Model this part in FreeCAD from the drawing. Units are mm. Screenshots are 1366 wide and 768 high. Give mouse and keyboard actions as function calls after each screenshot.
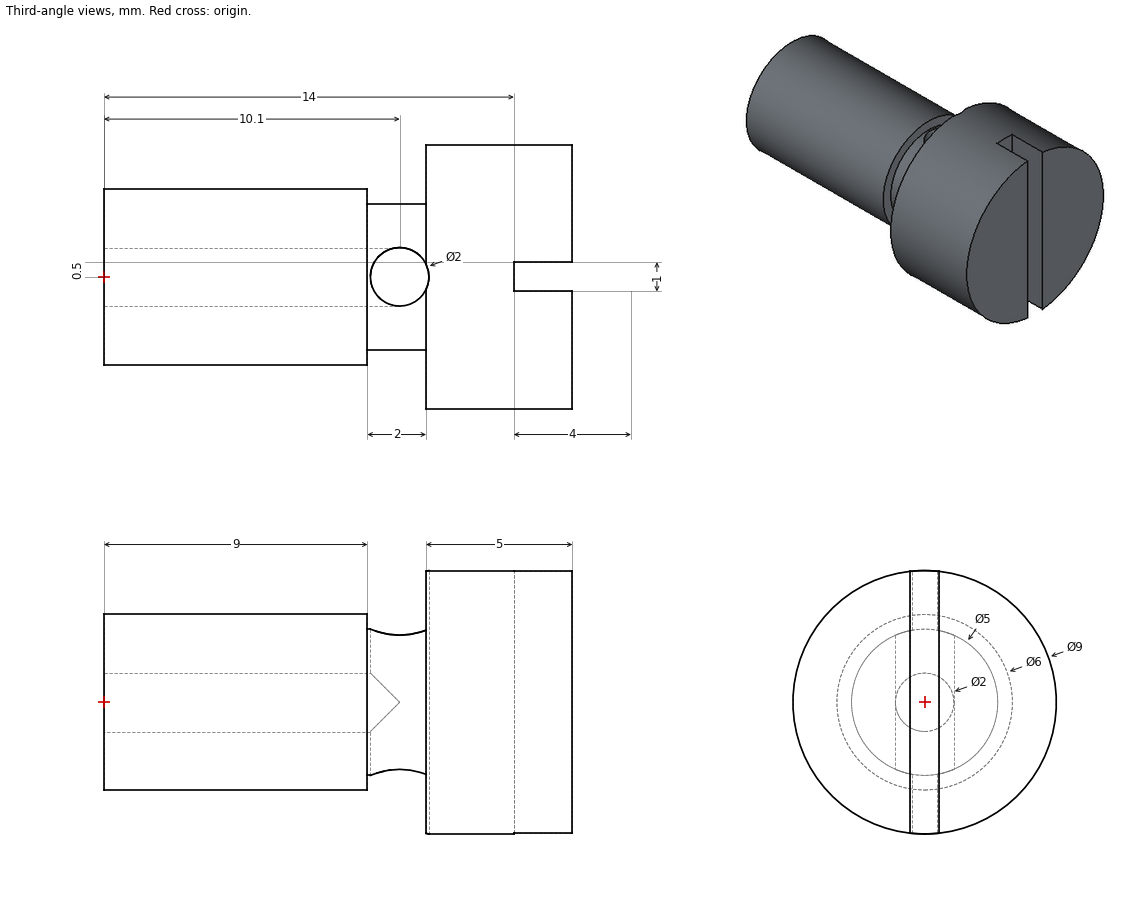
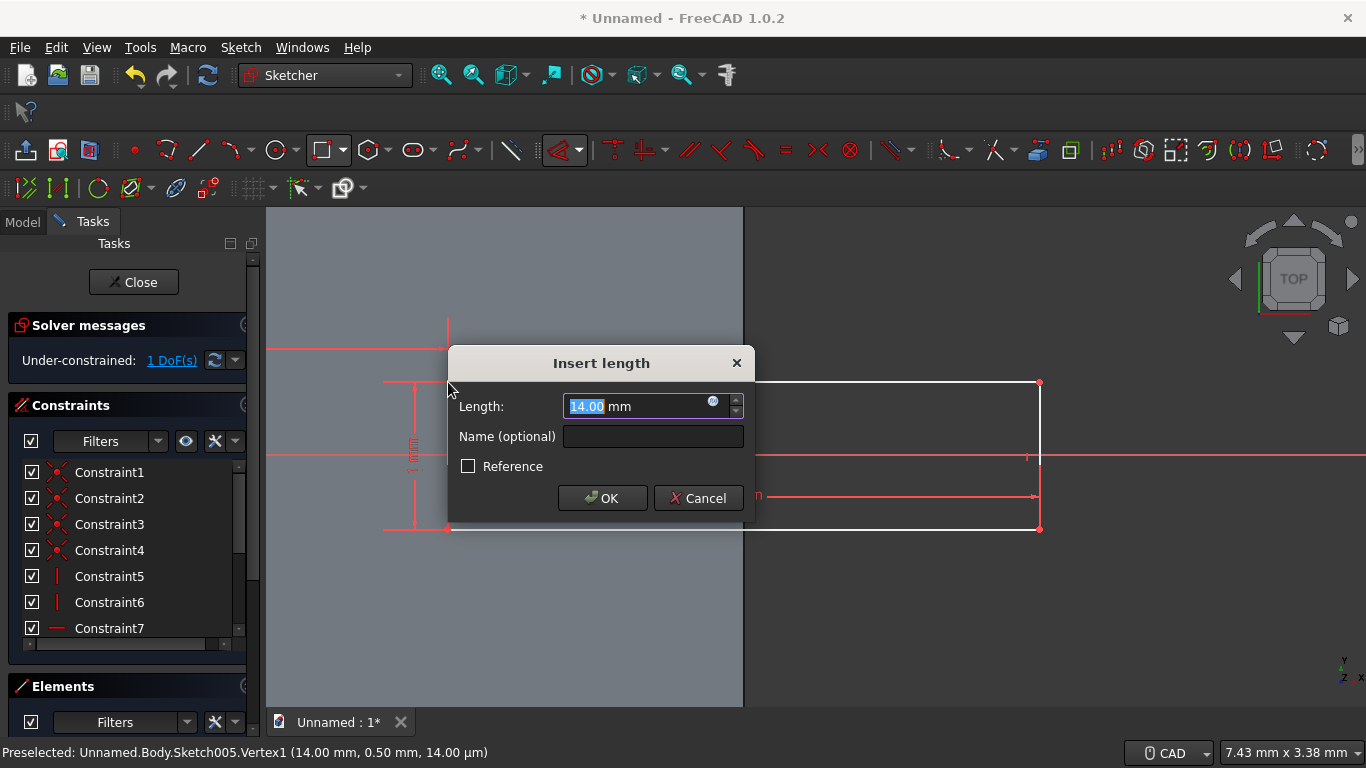
text(14)
key(Return)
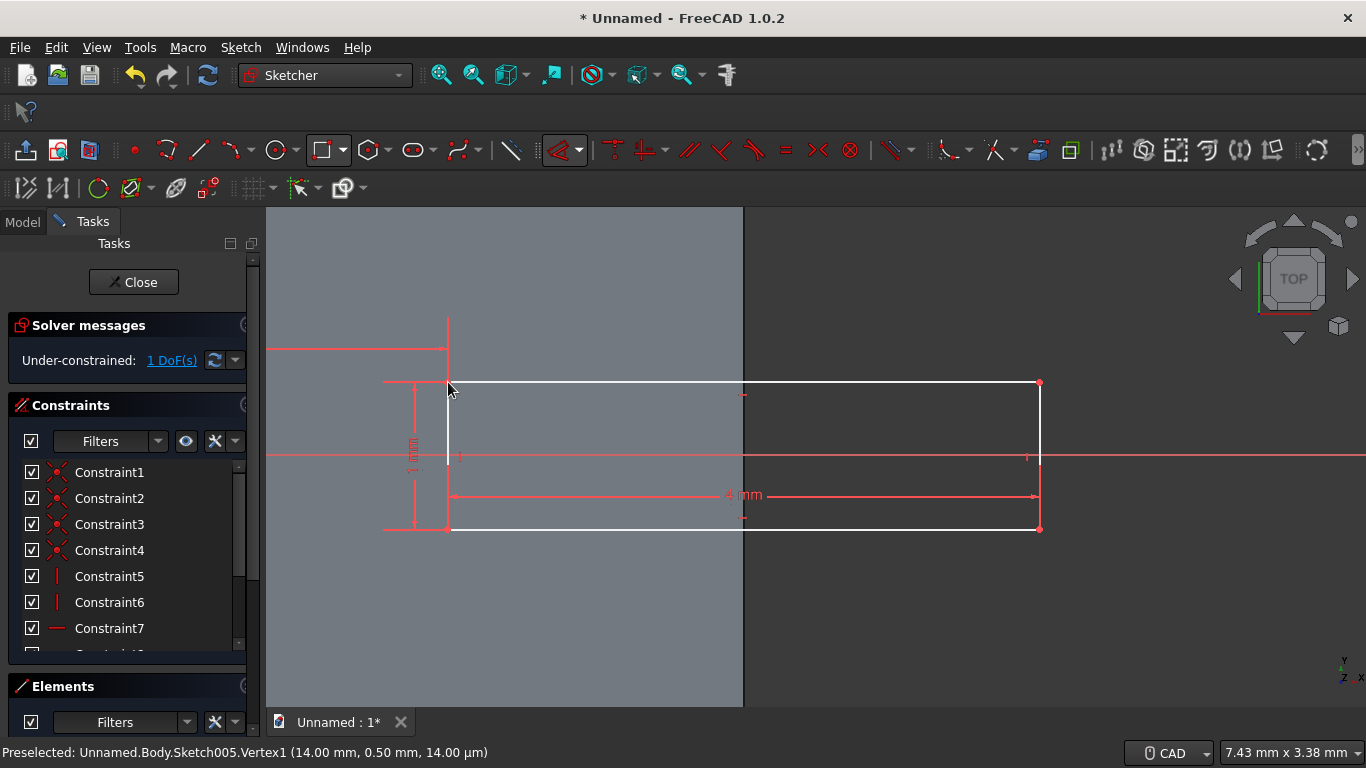
click(448, 382)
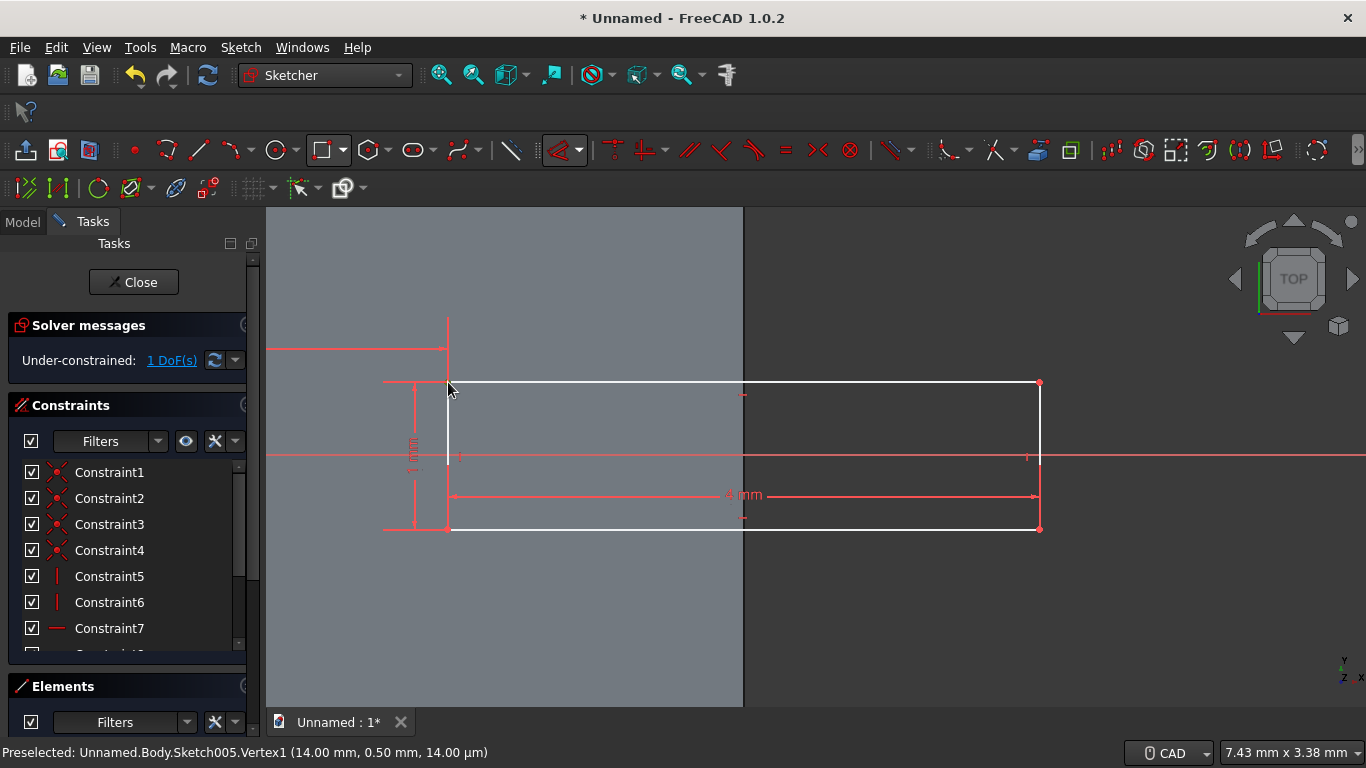
click(582, 150)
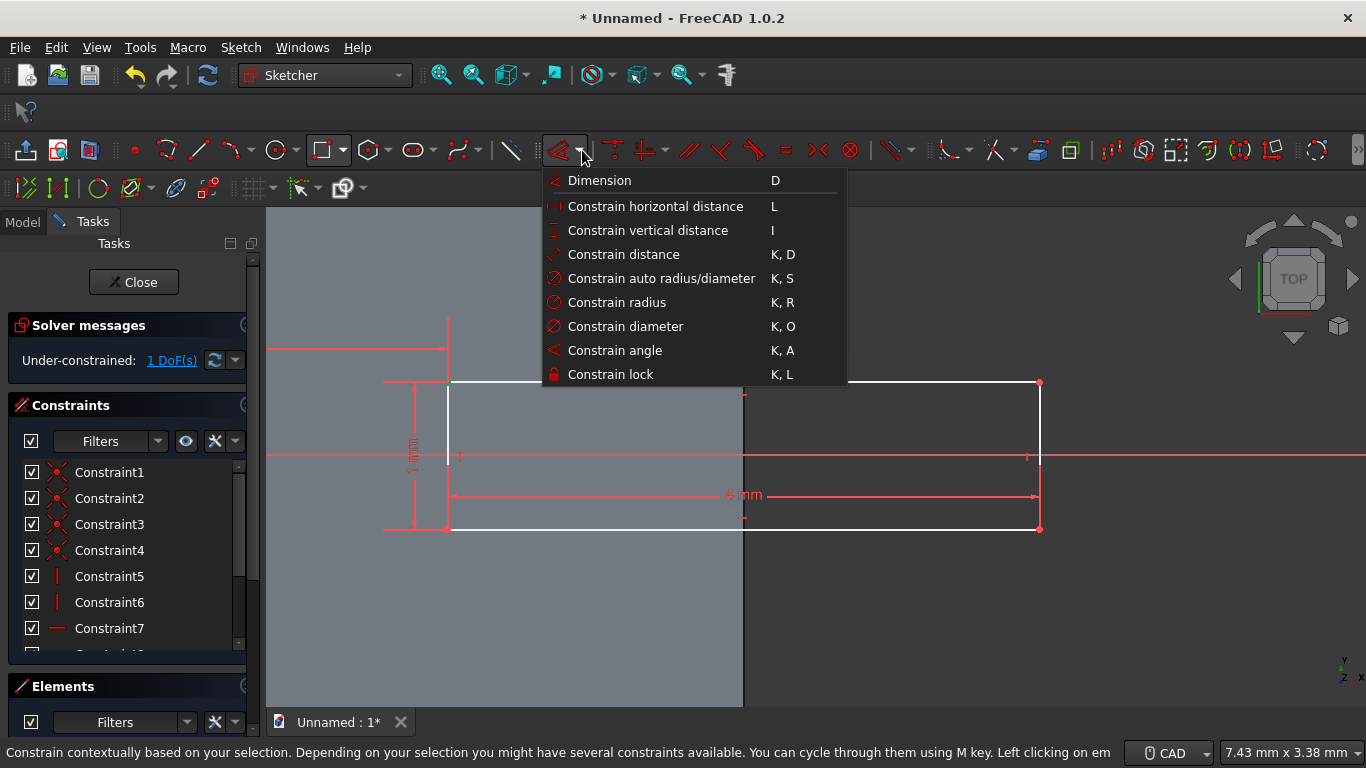
click(695, 230)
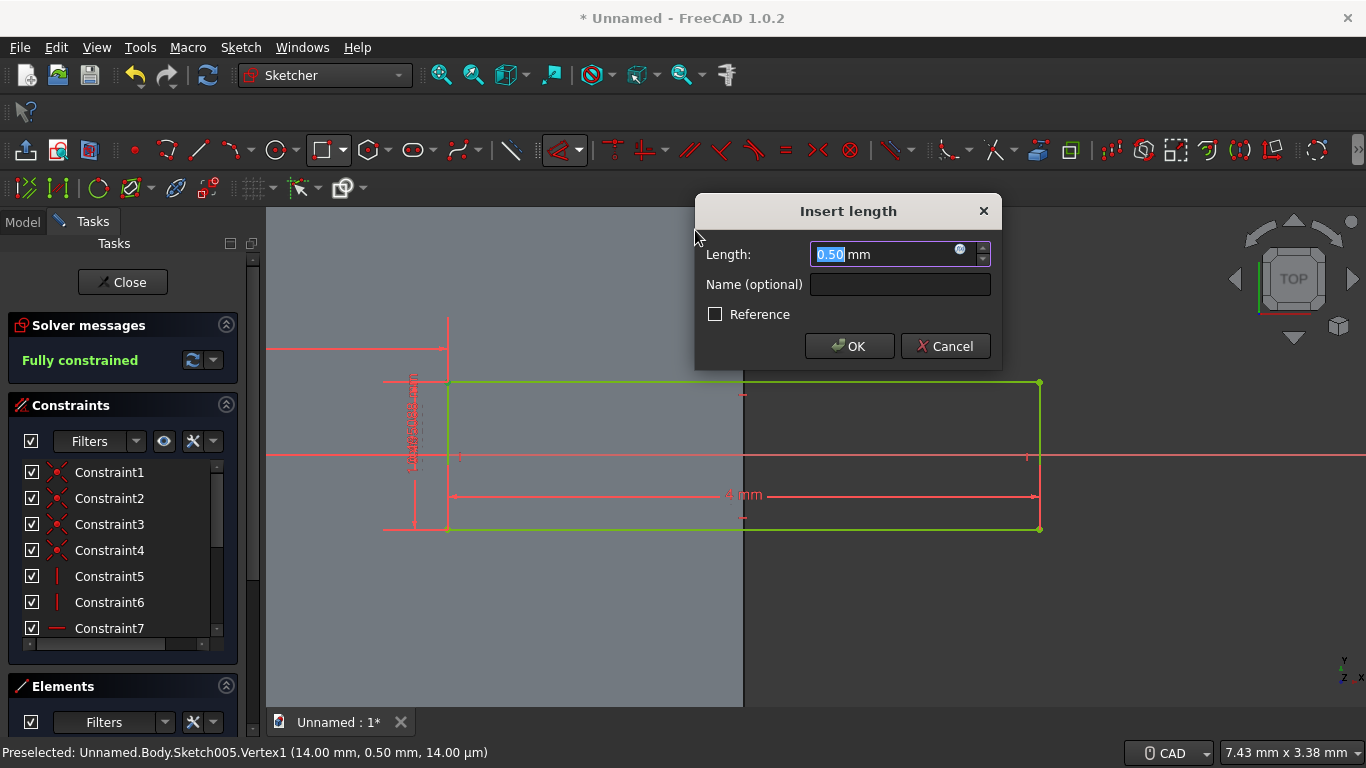
text(0.5)
key(Return)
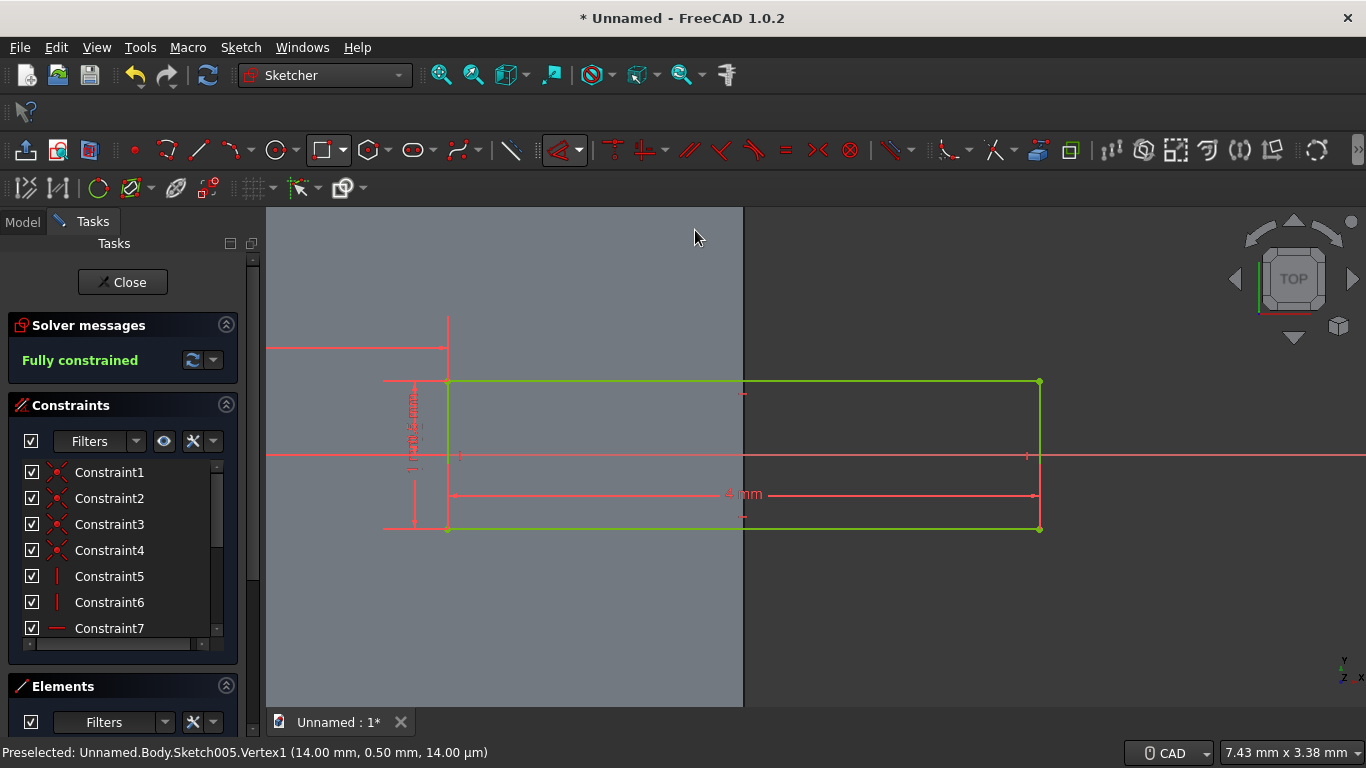
click(123, 282)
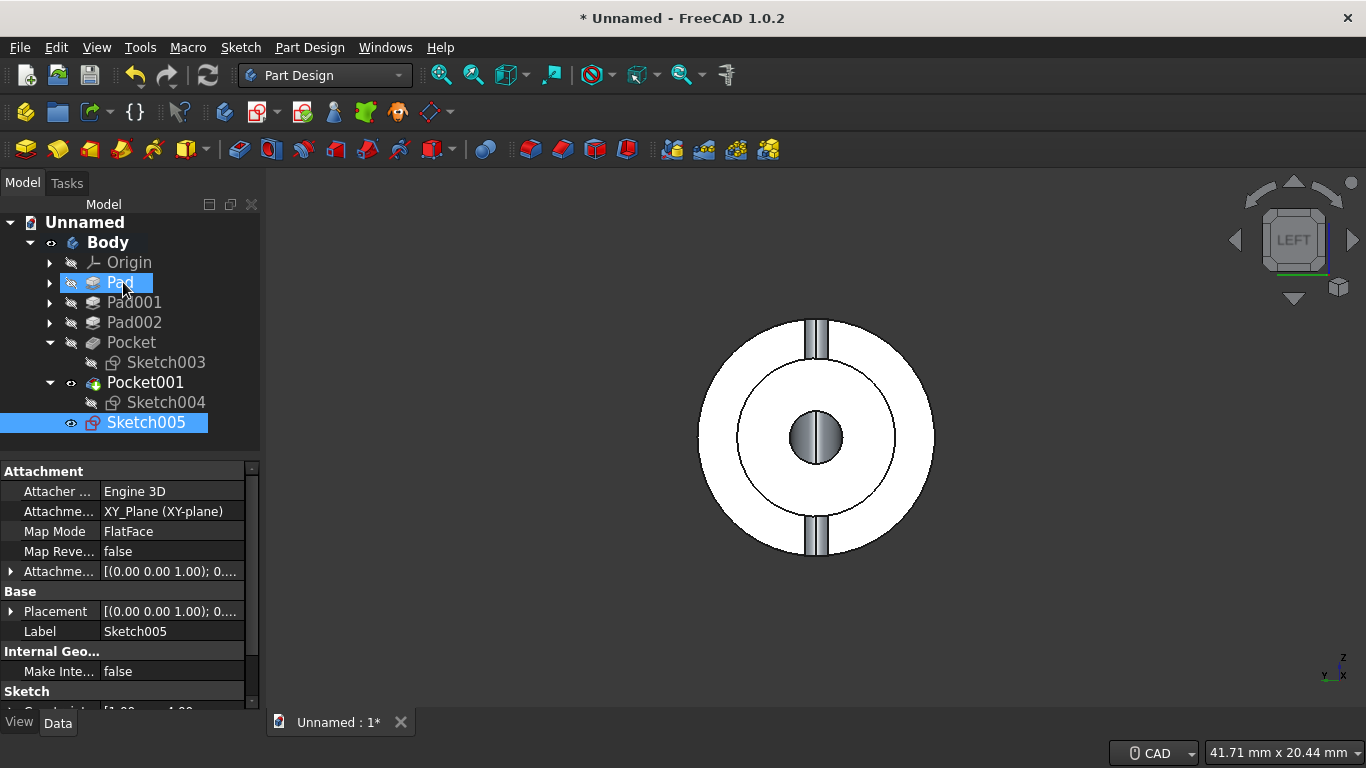
click(240, 150)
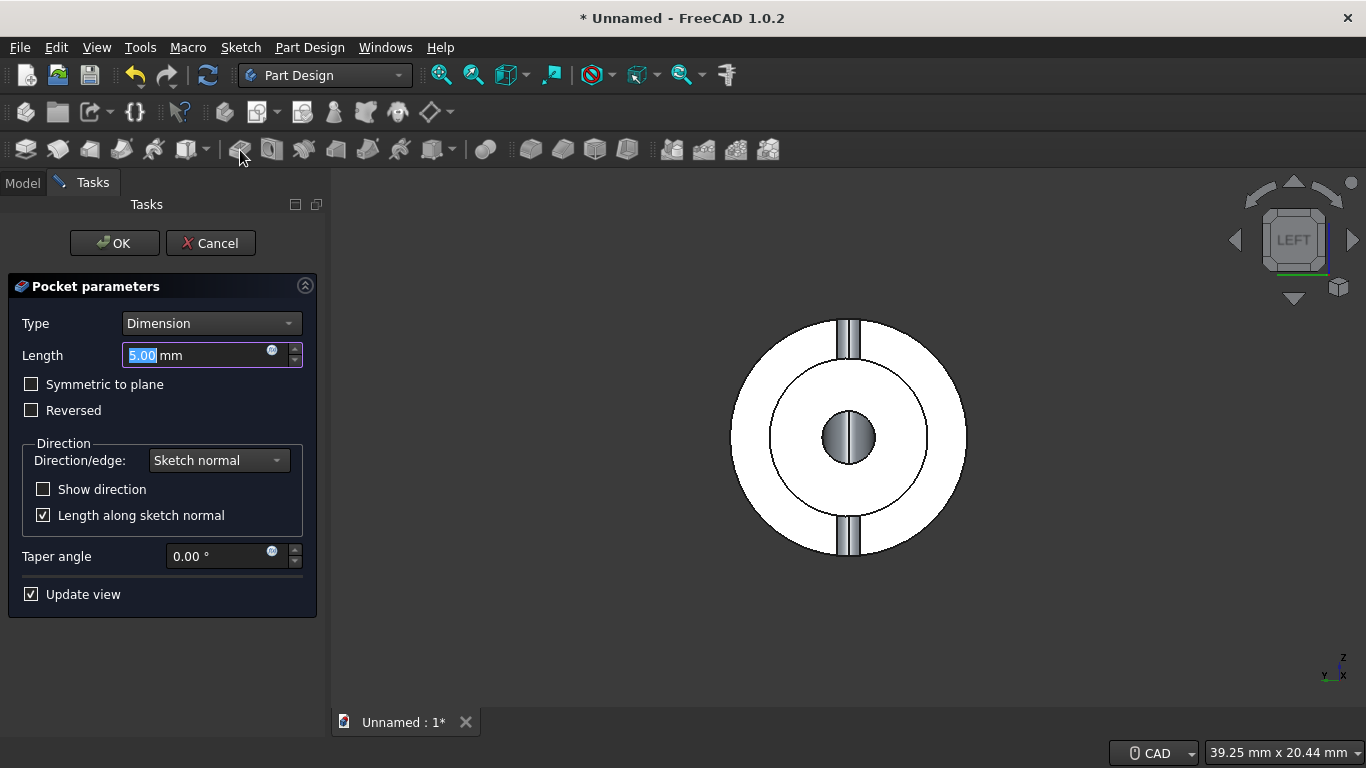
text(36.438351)
key(Tab)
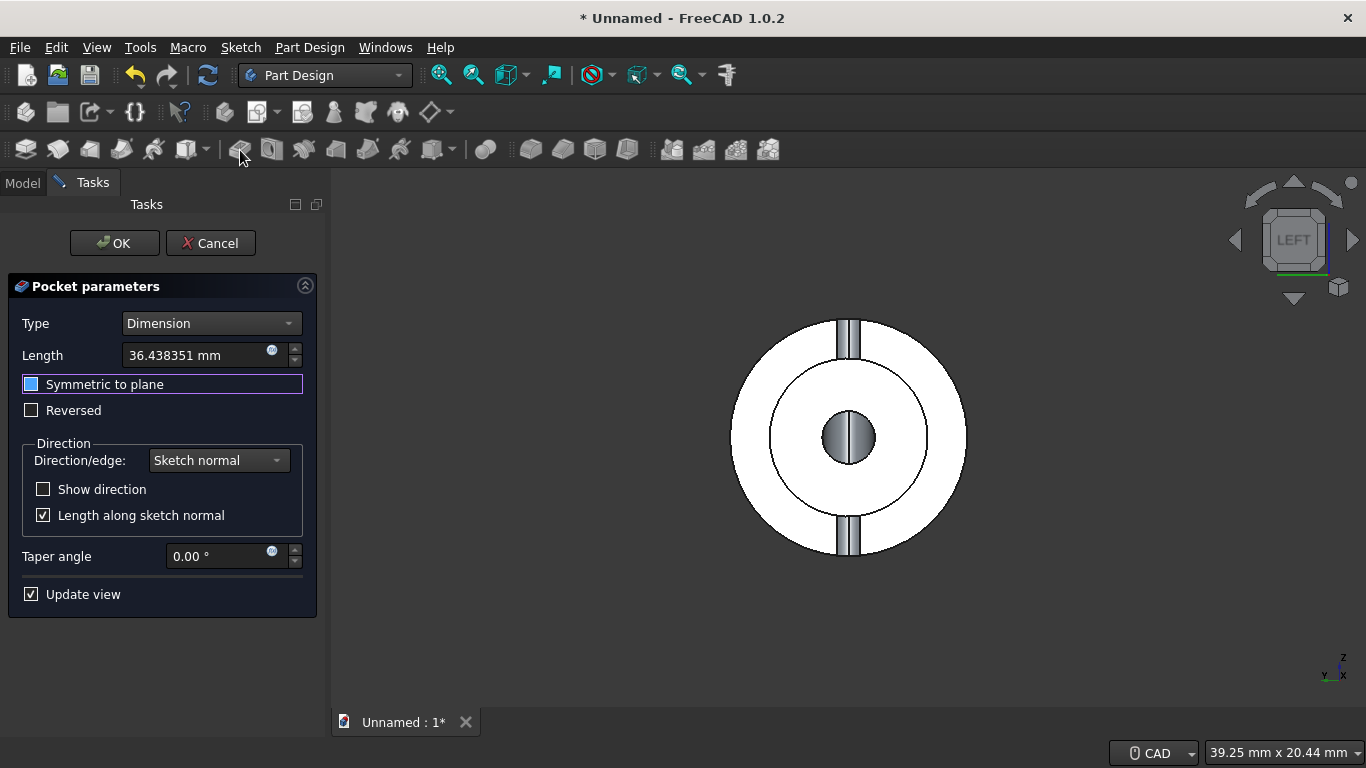
click(30, 384)